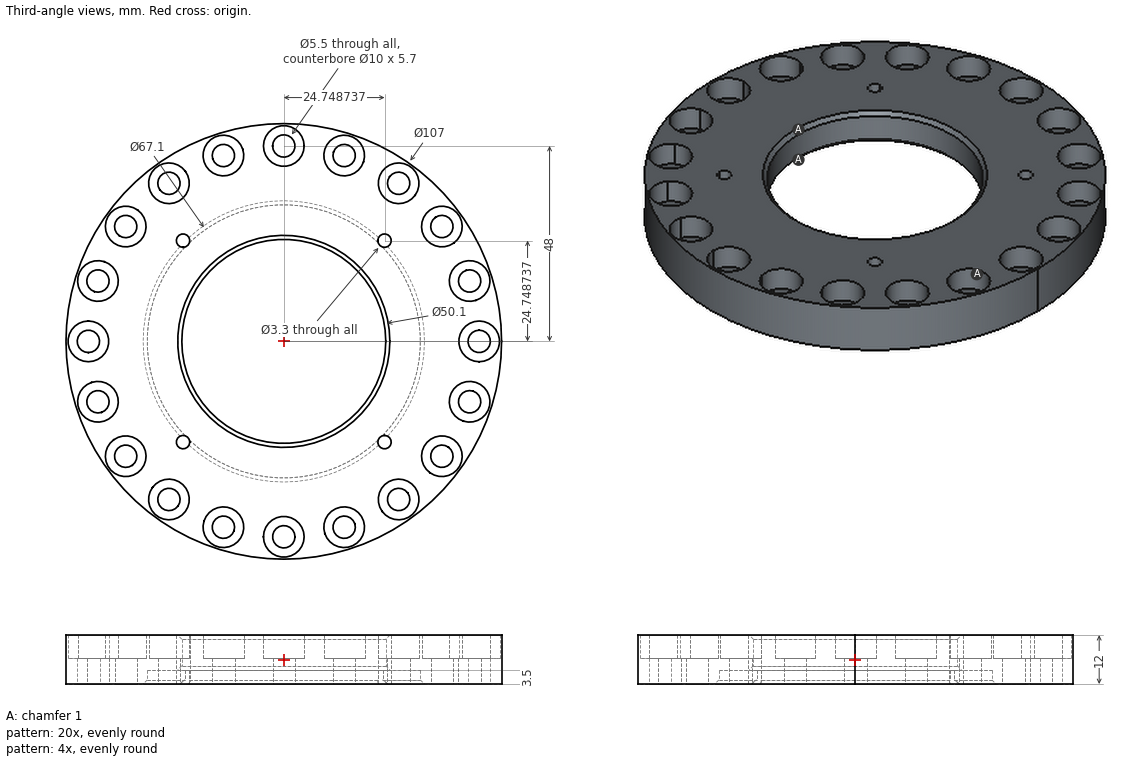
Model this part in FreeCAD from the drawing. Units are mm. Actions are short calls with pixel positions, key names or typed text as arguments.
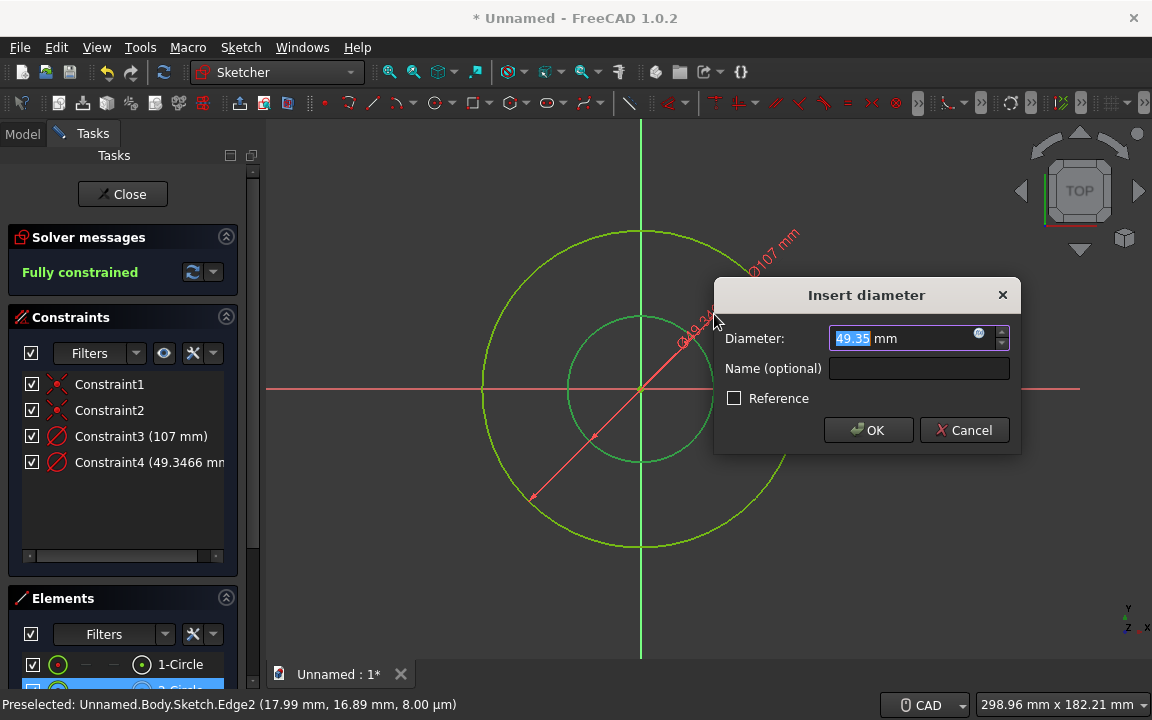
text(50.1)
key(Return)
key(Escape)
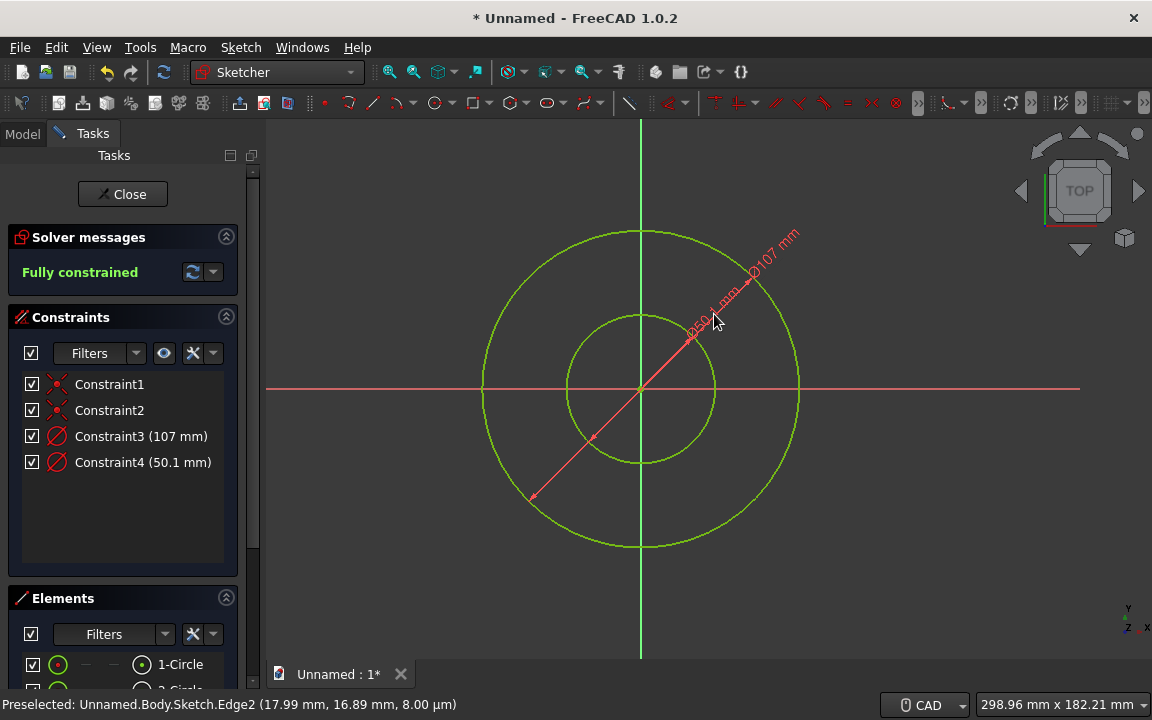
click(123, 194)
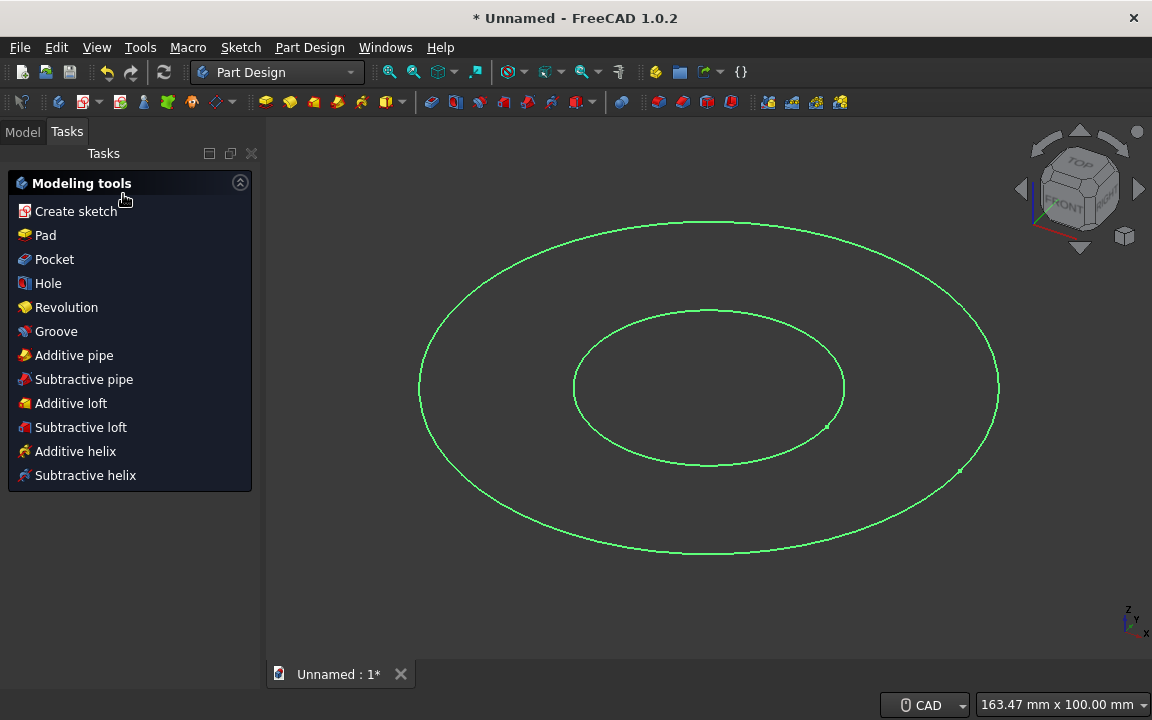
click(266, 102)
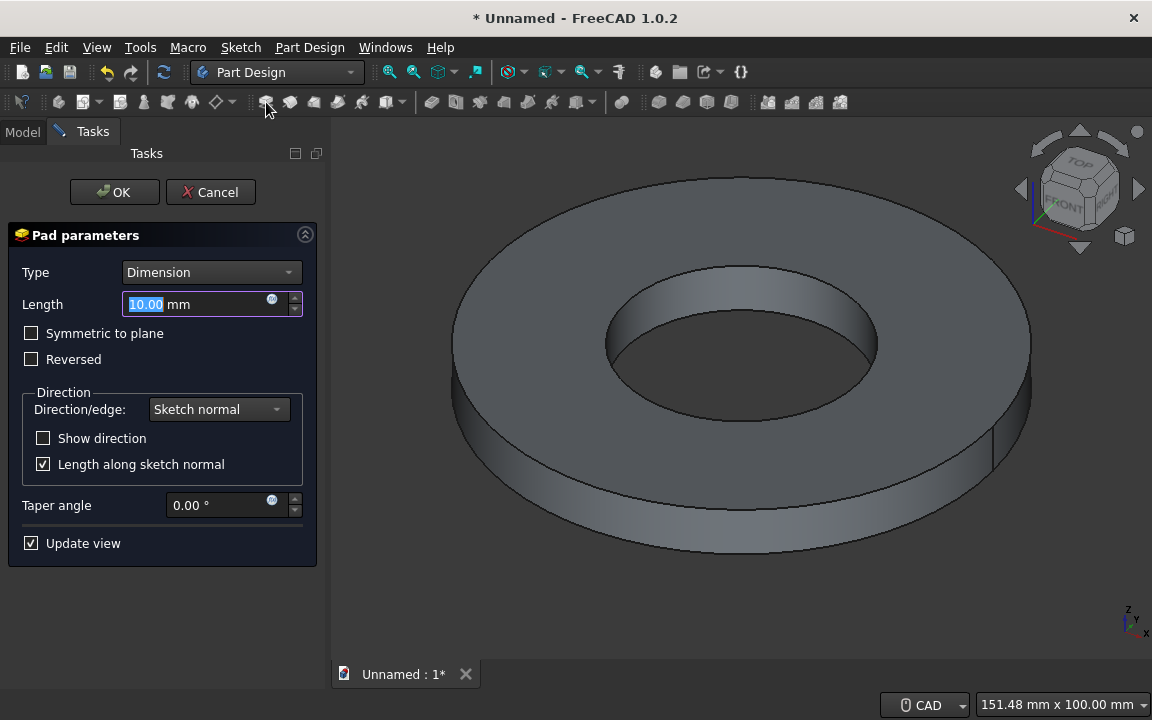
text(12)
key(Tab)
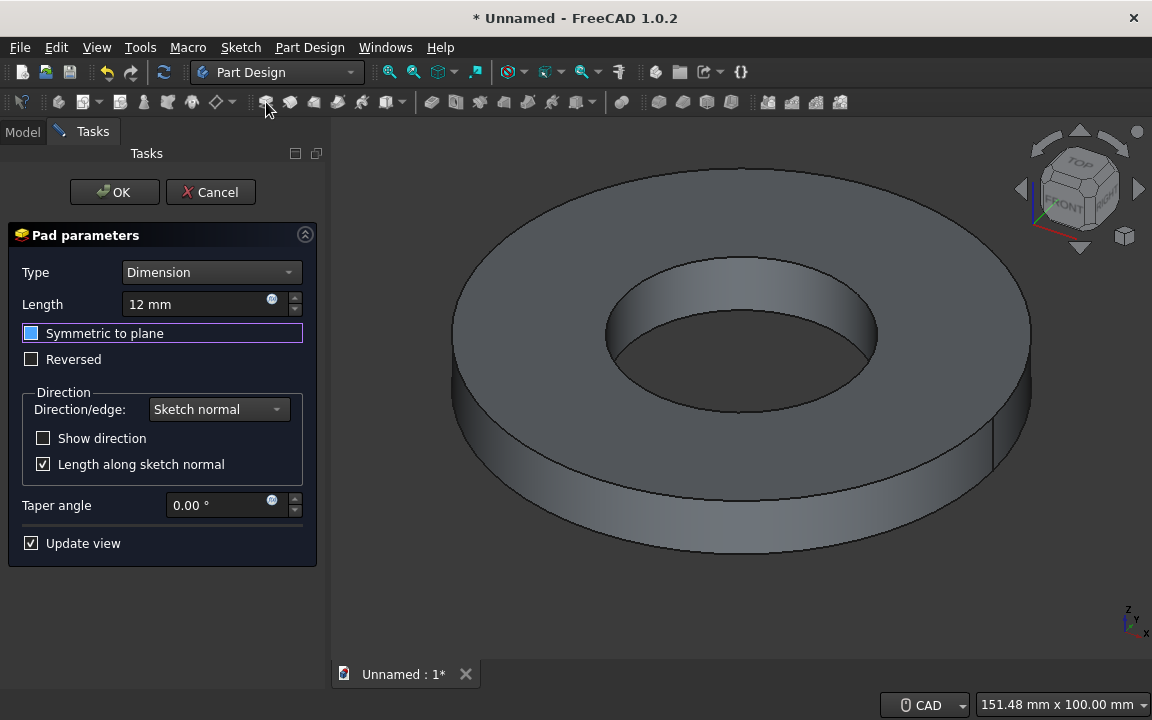
click(30, 333)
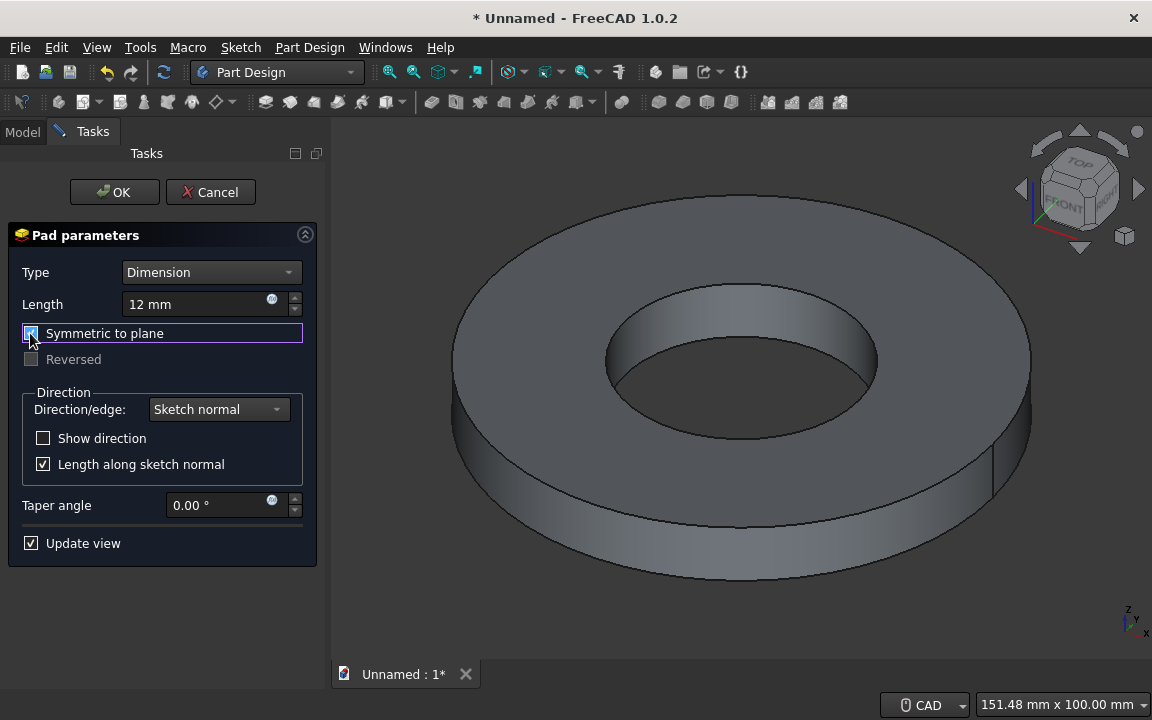
click(115, 192)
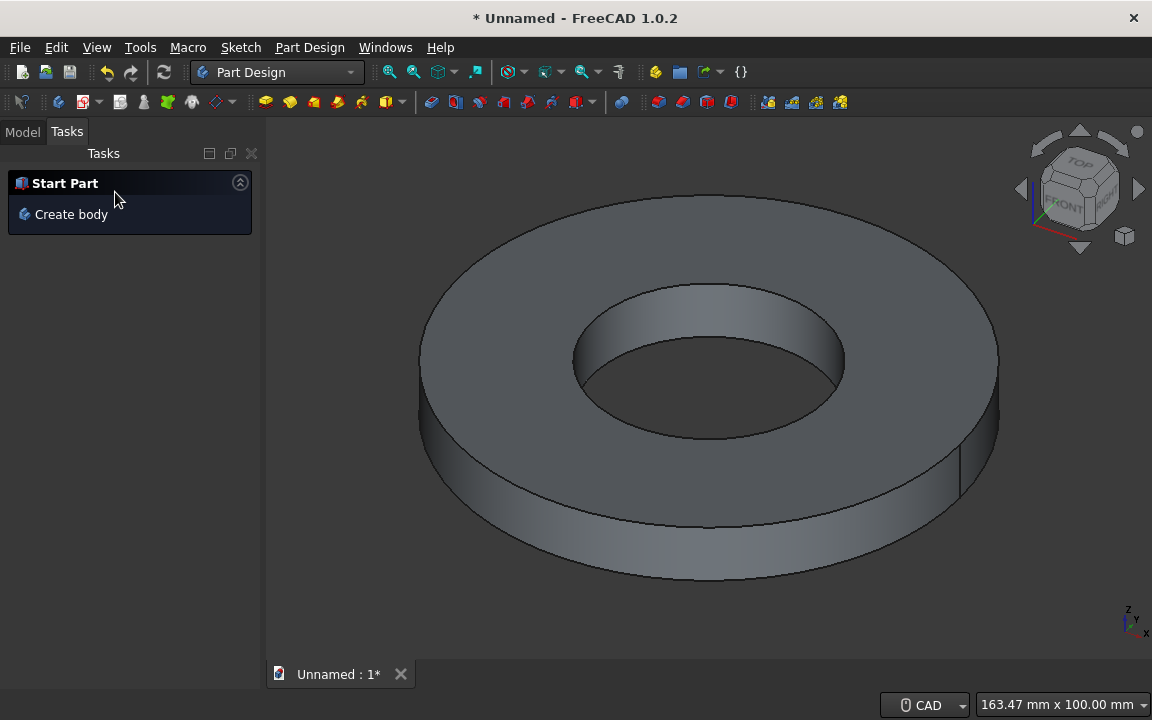
click(935, 326)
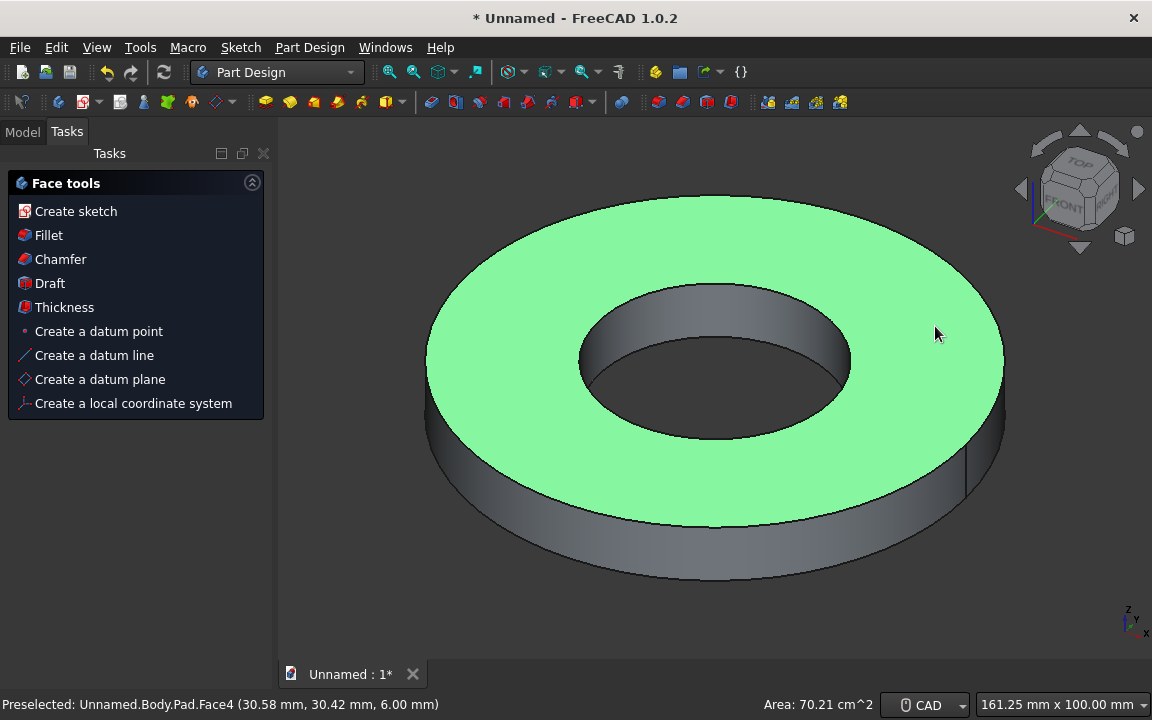
click(84, 102)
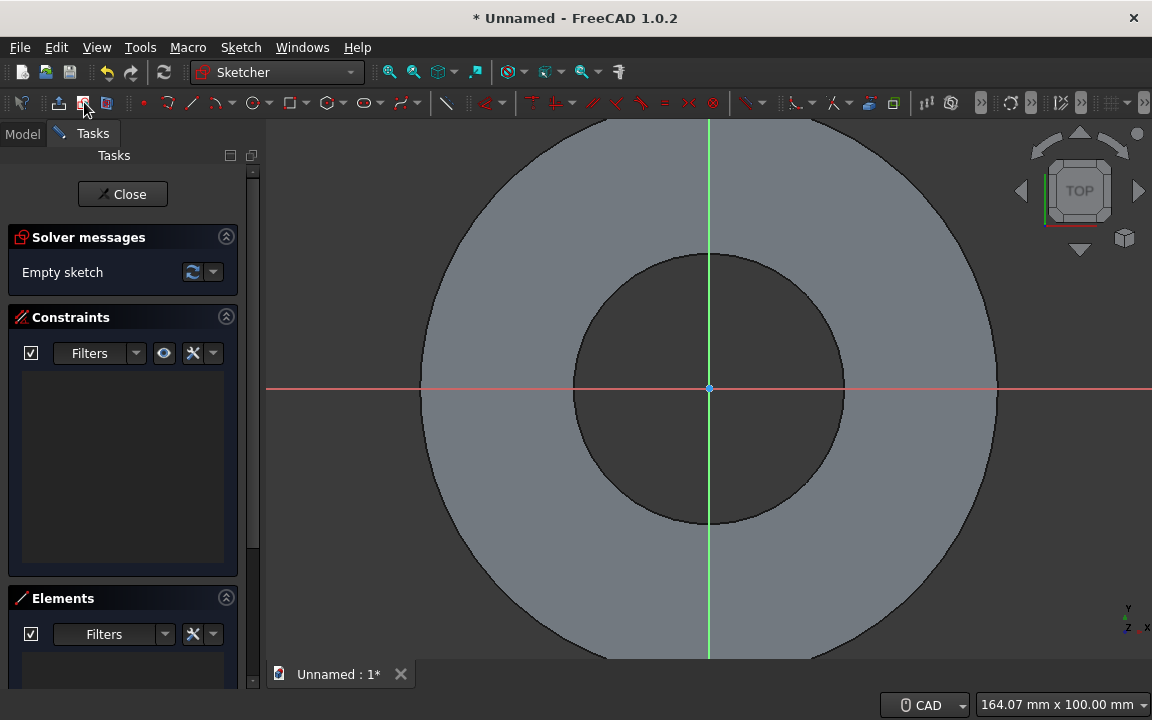
scroll(640, 389, down, 5)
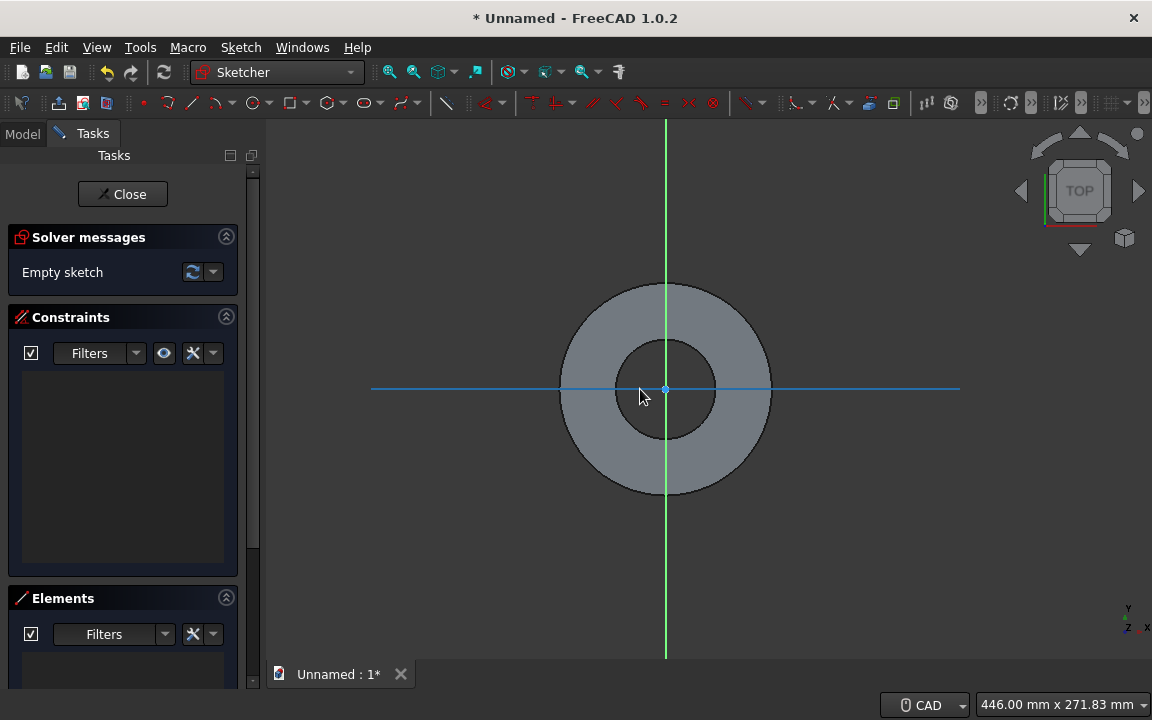
scroll(667, 289, up, 15)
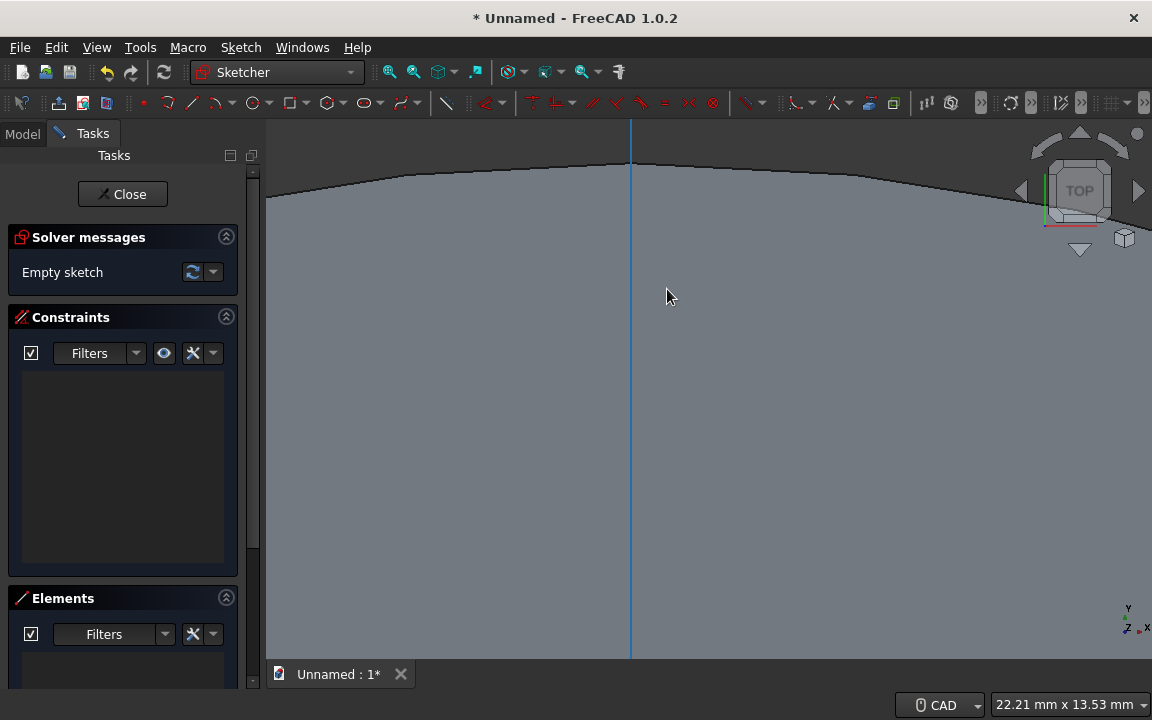
scroll(612, 370, up, 2)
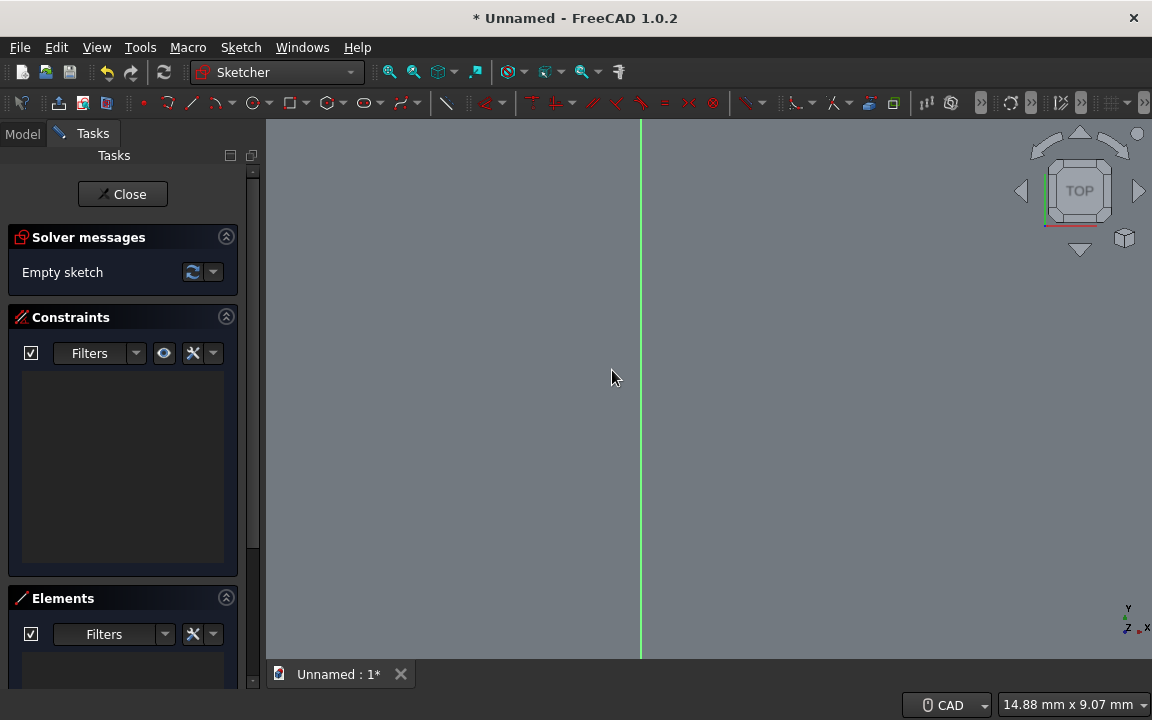
click(254, 104)